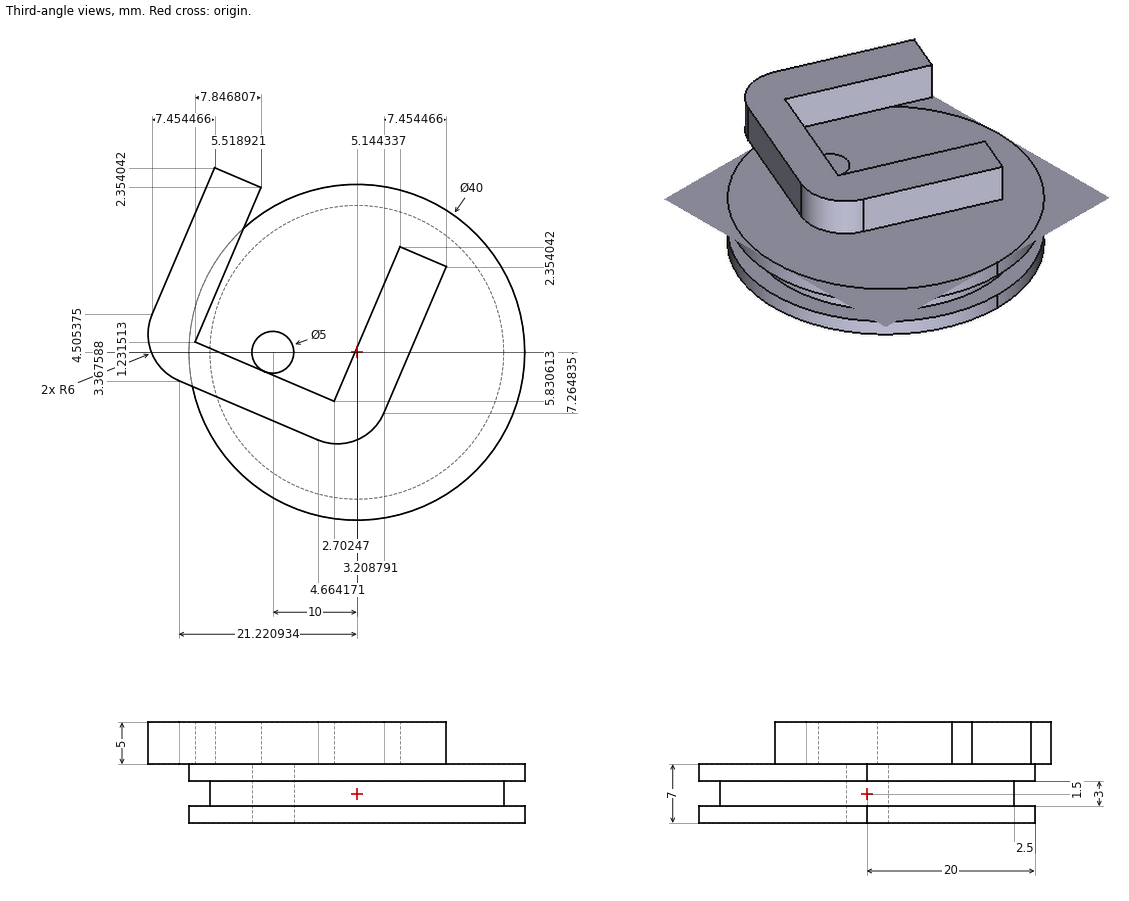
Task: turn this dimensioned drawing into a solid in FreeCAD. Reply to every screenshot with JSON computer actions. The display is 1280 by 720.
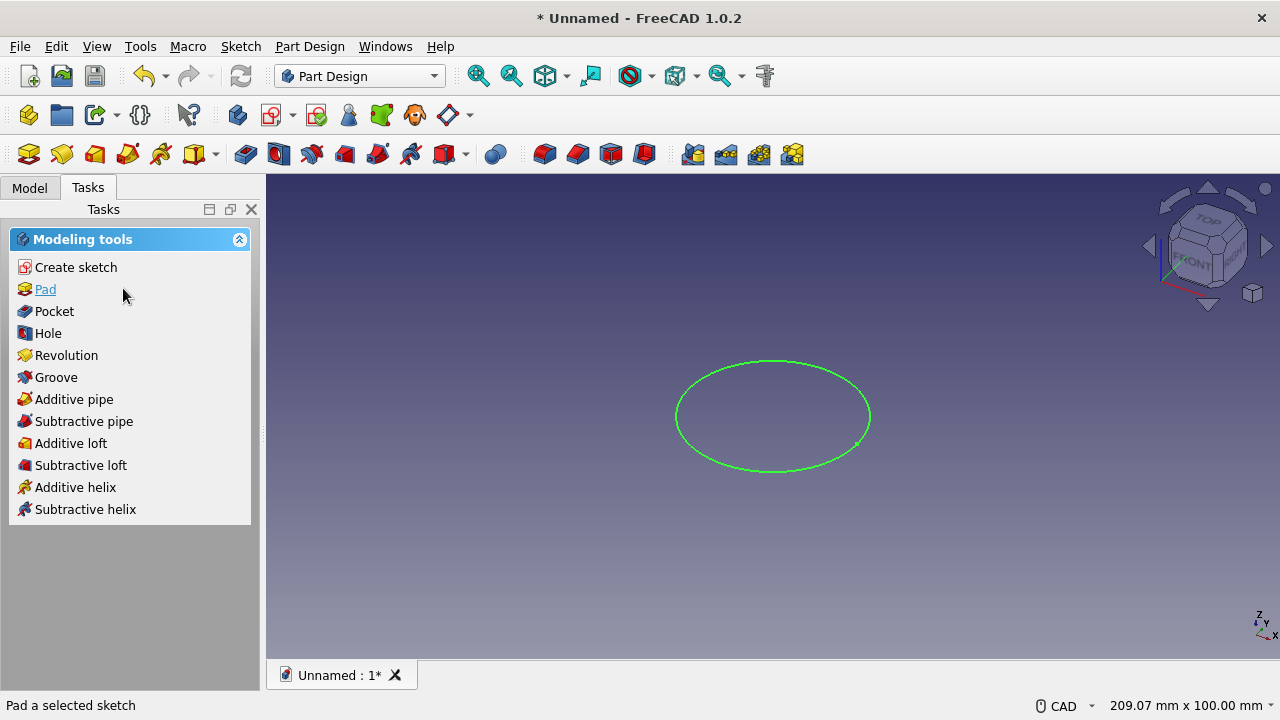
{"action": "left_click", "coordinate": [29, 154]}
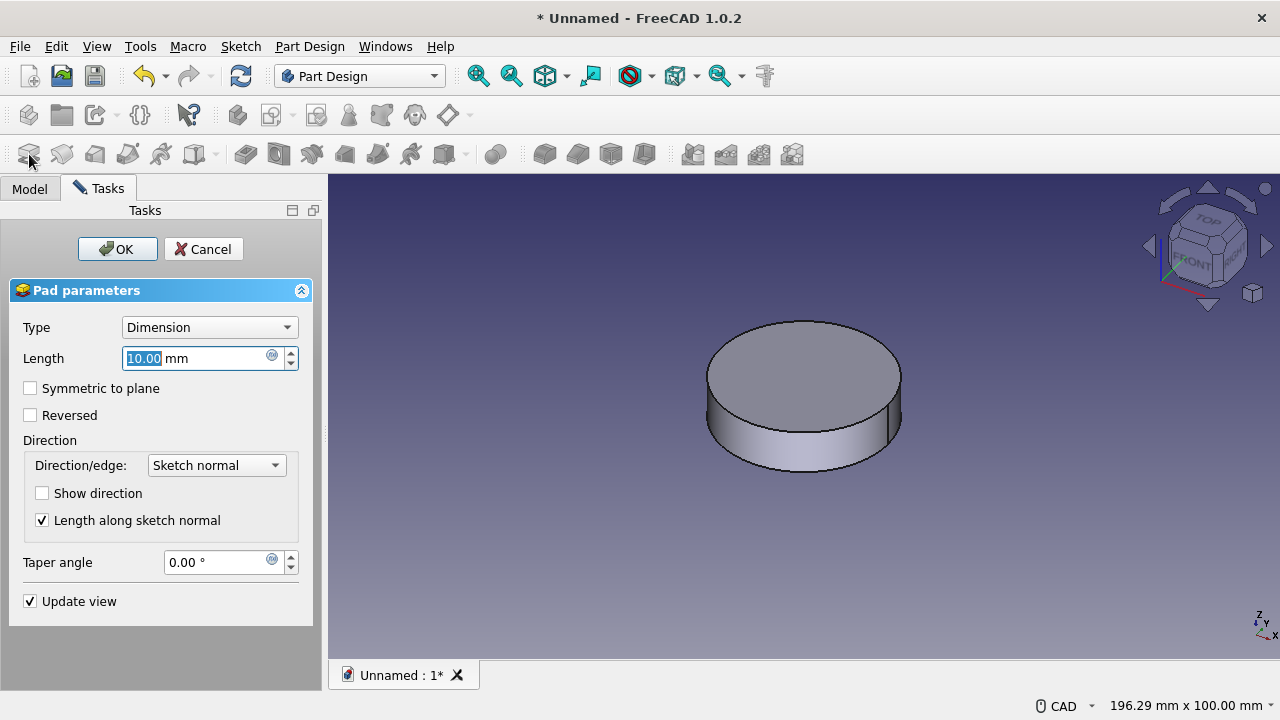
{"action": "type", "text": "7"}
{"action": "key", "text": "Tab"}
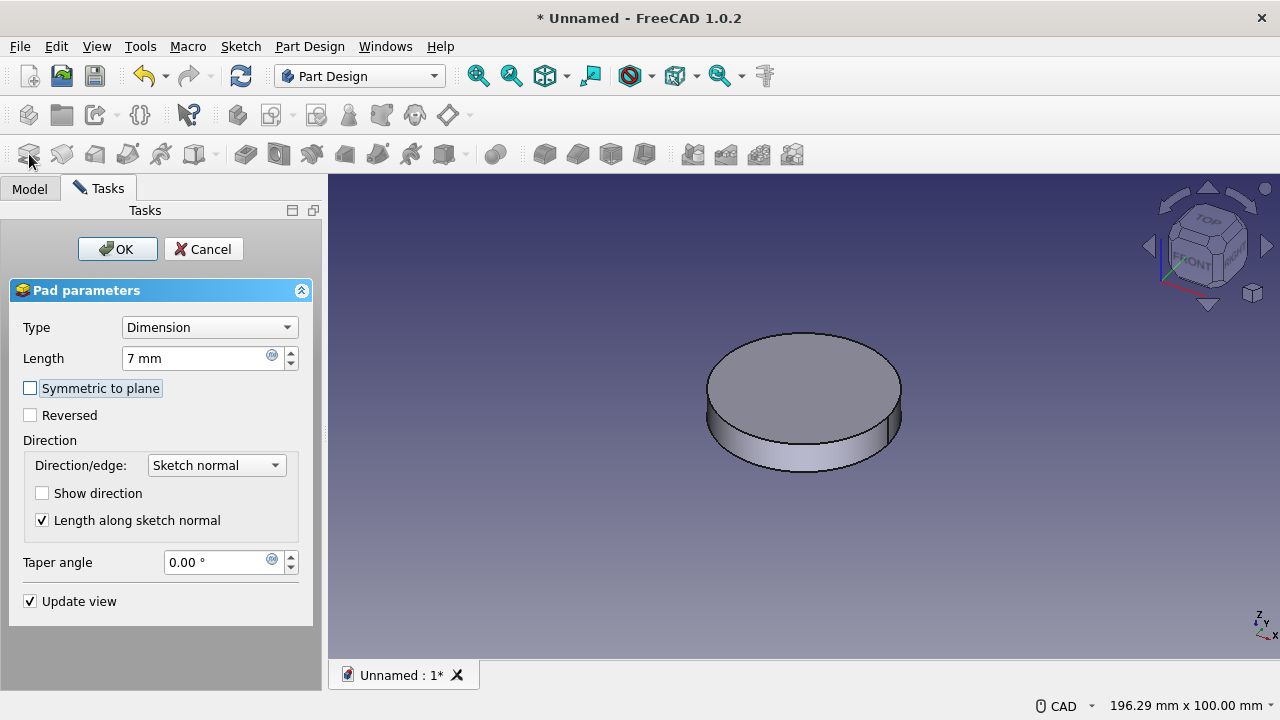
{"action": "left_click", "coordinate": [31, 388]}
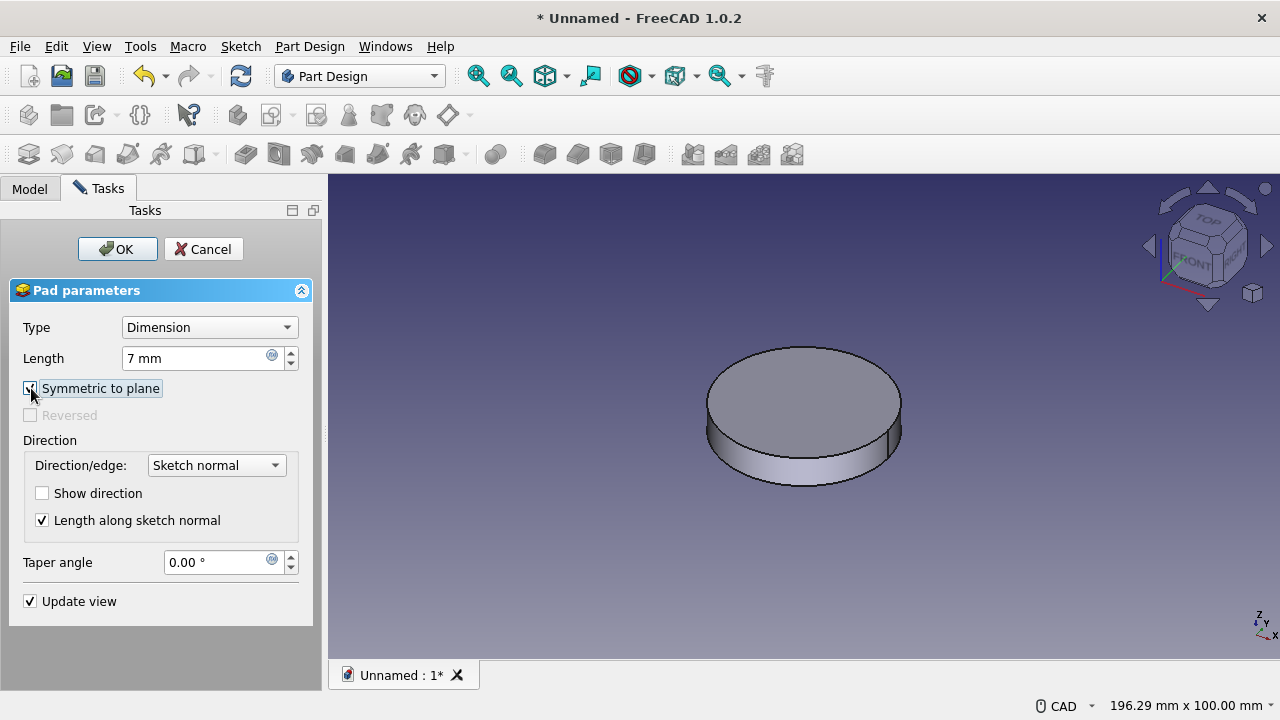
{"action": "left_click", "coordinate": [118, 249]}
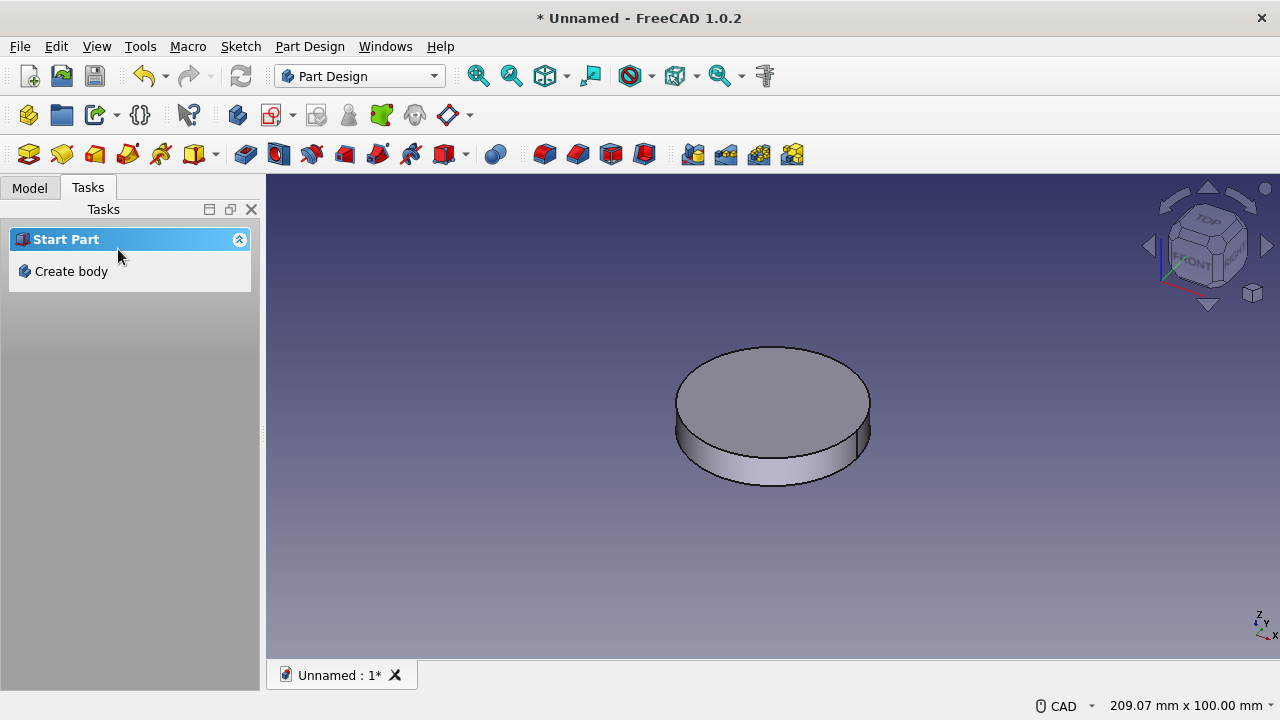
{"action": "left_click", "coordinate": [479, 76]}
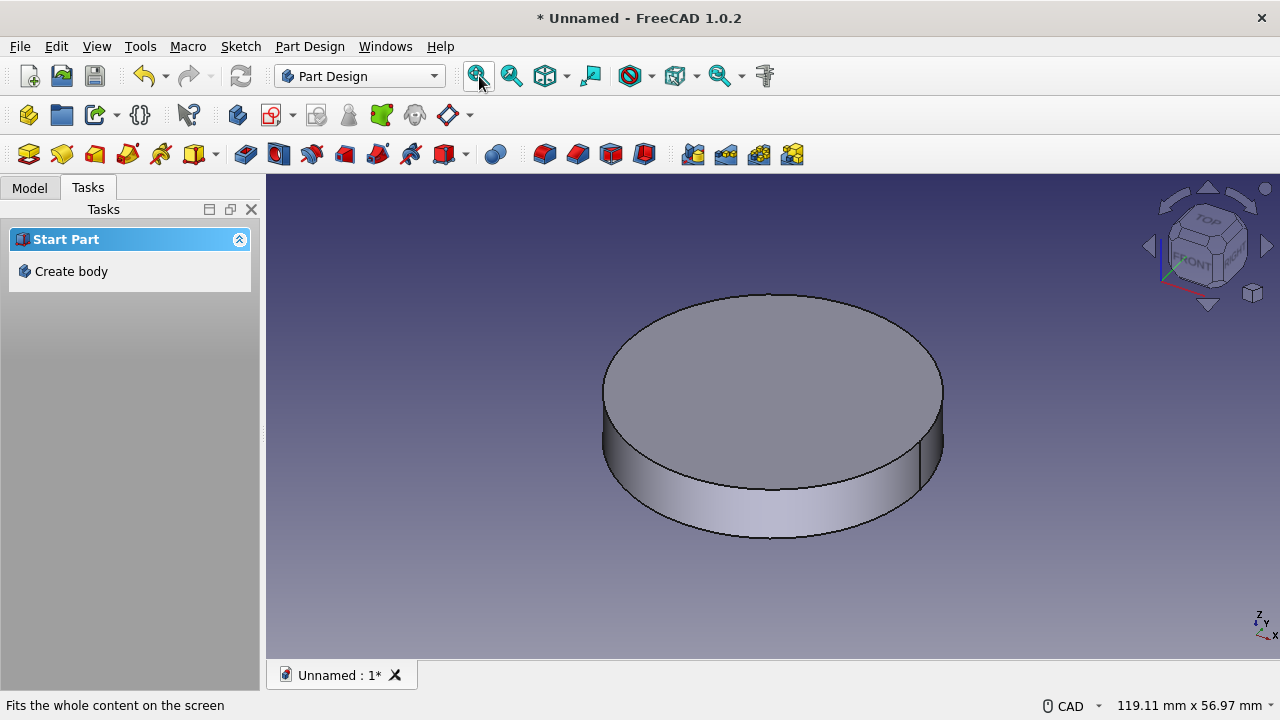
{"action": "left_click", "coordinate": [270, 116]}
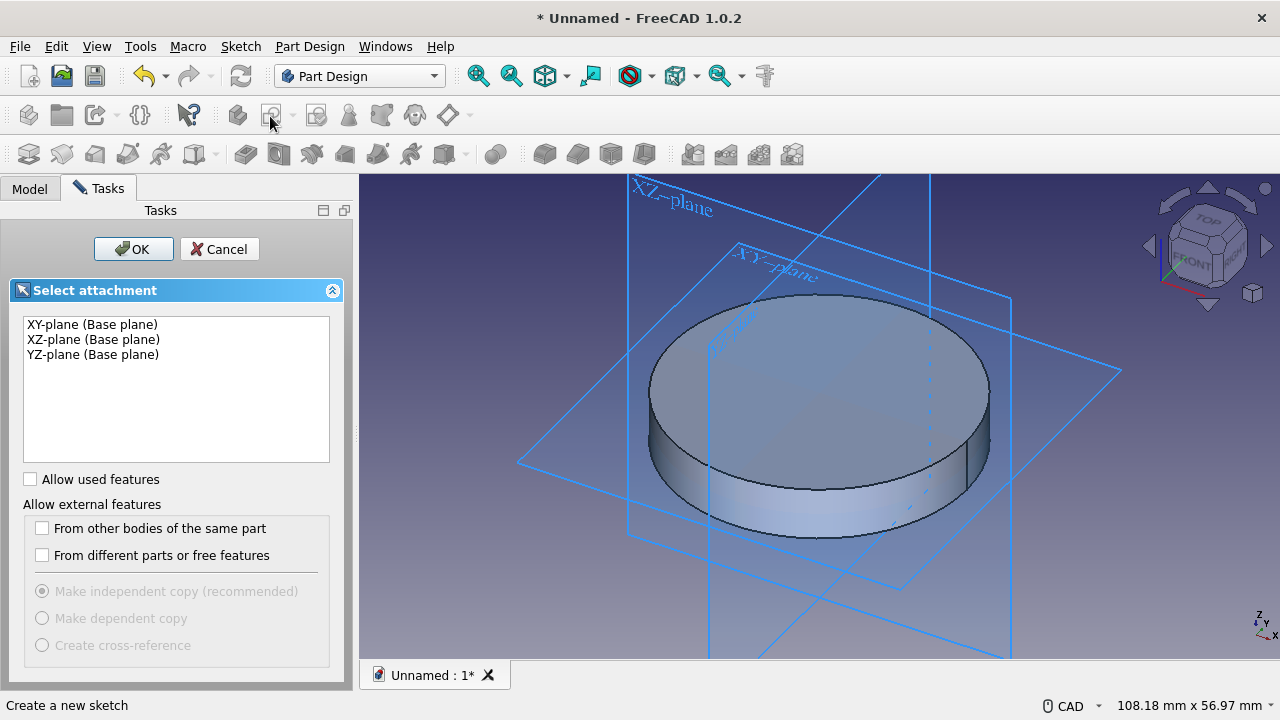
{"action": "left_click", "coordinate": [84, 354]}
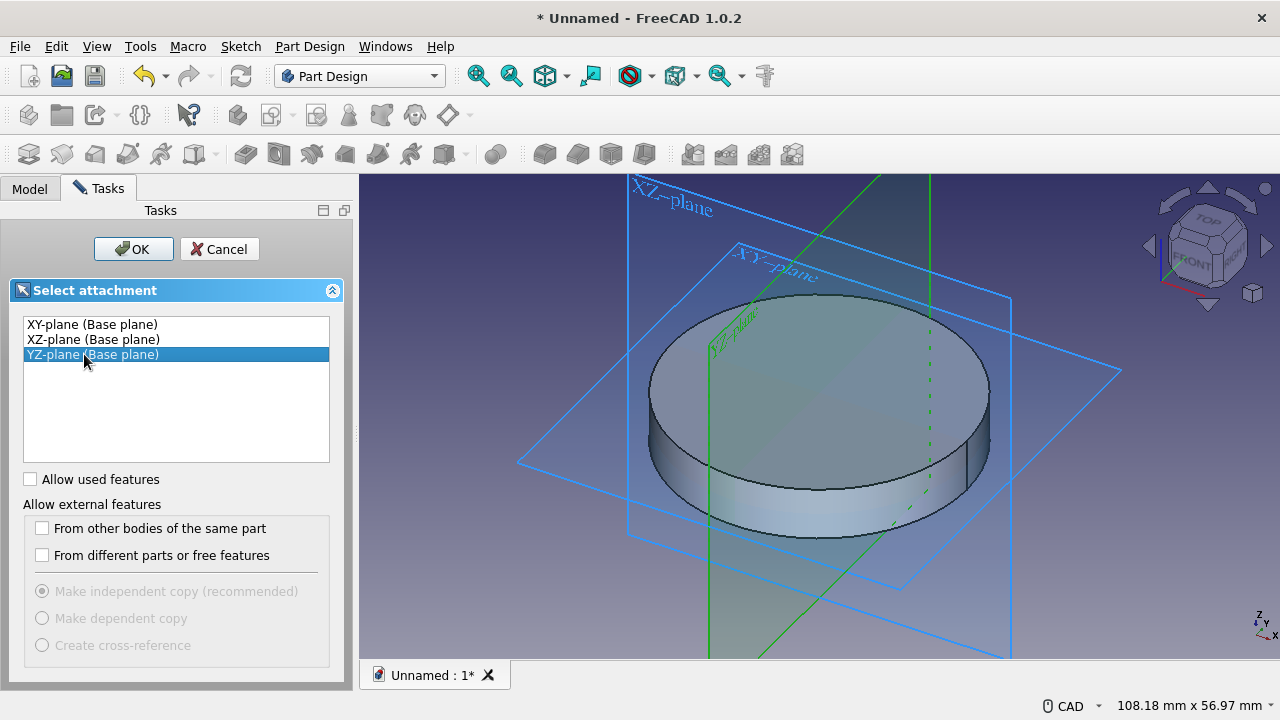
{"action": "left_click", "coordinate": [134, 249]}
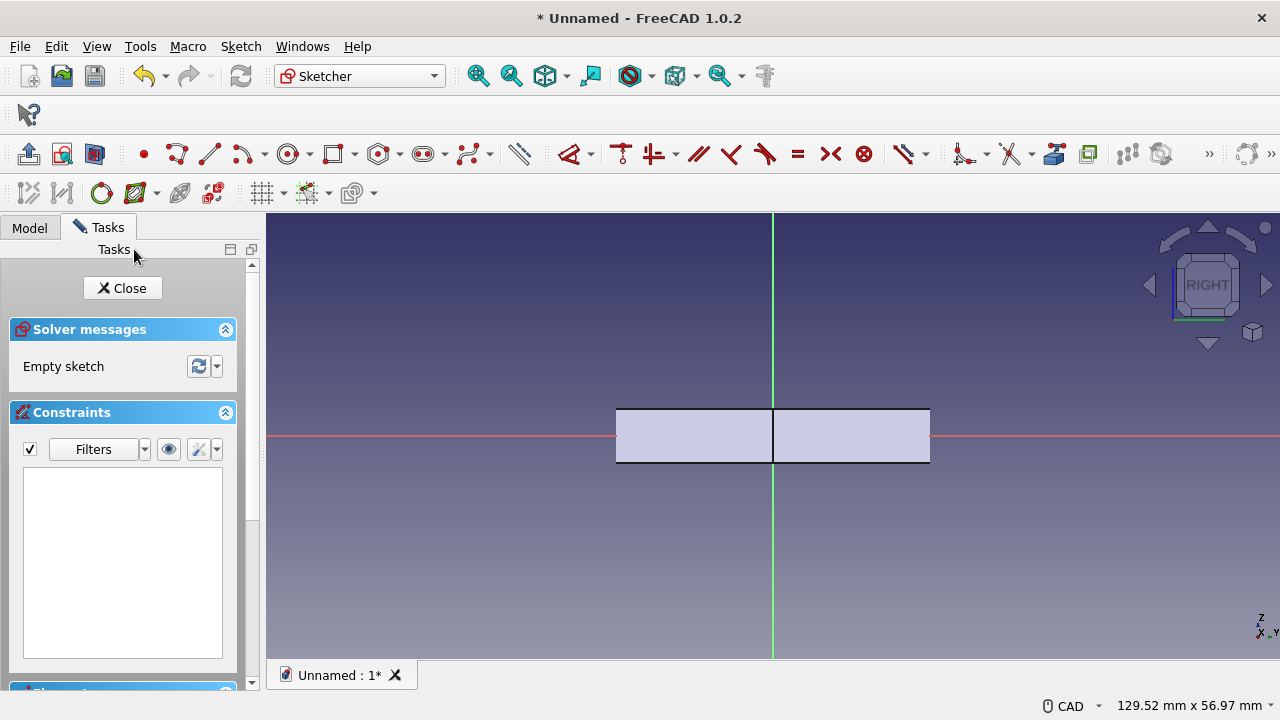
{"action": "left_click", "coordinate": [95, 154]}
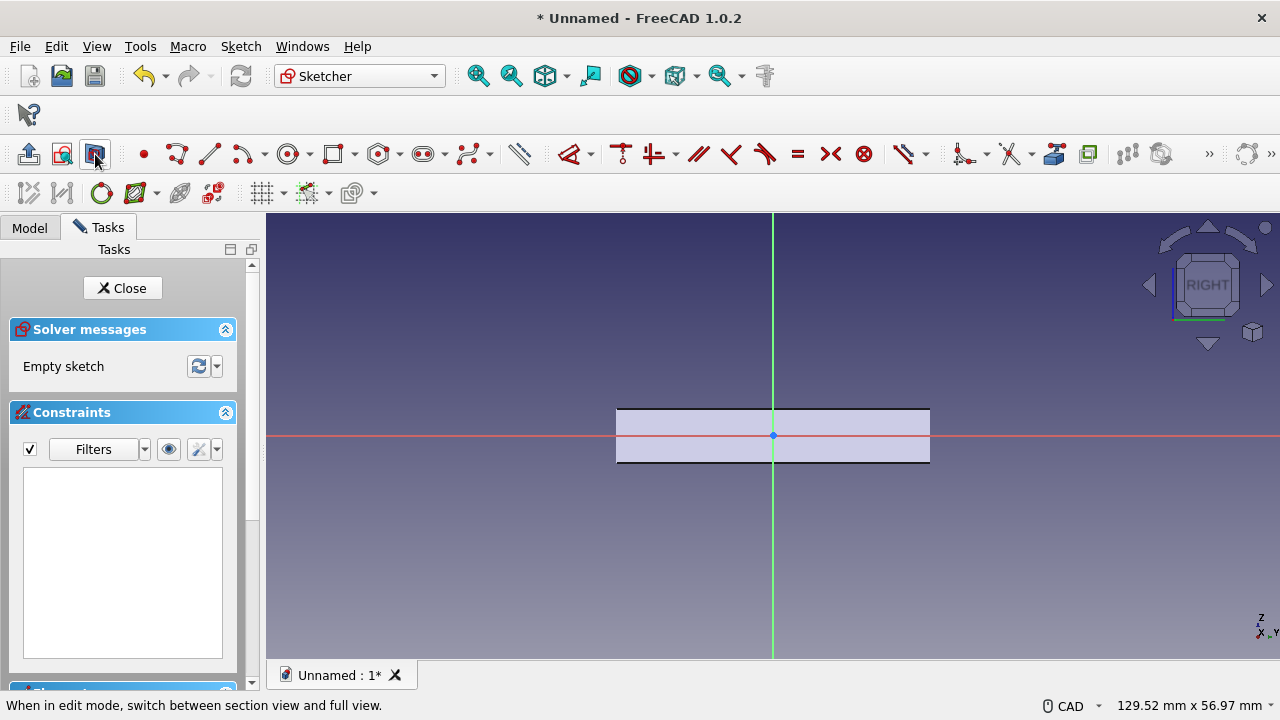
{"action": "scroll", "coordinate": [941, 436], "scroll_direction": "up", "scroll_amount": 12}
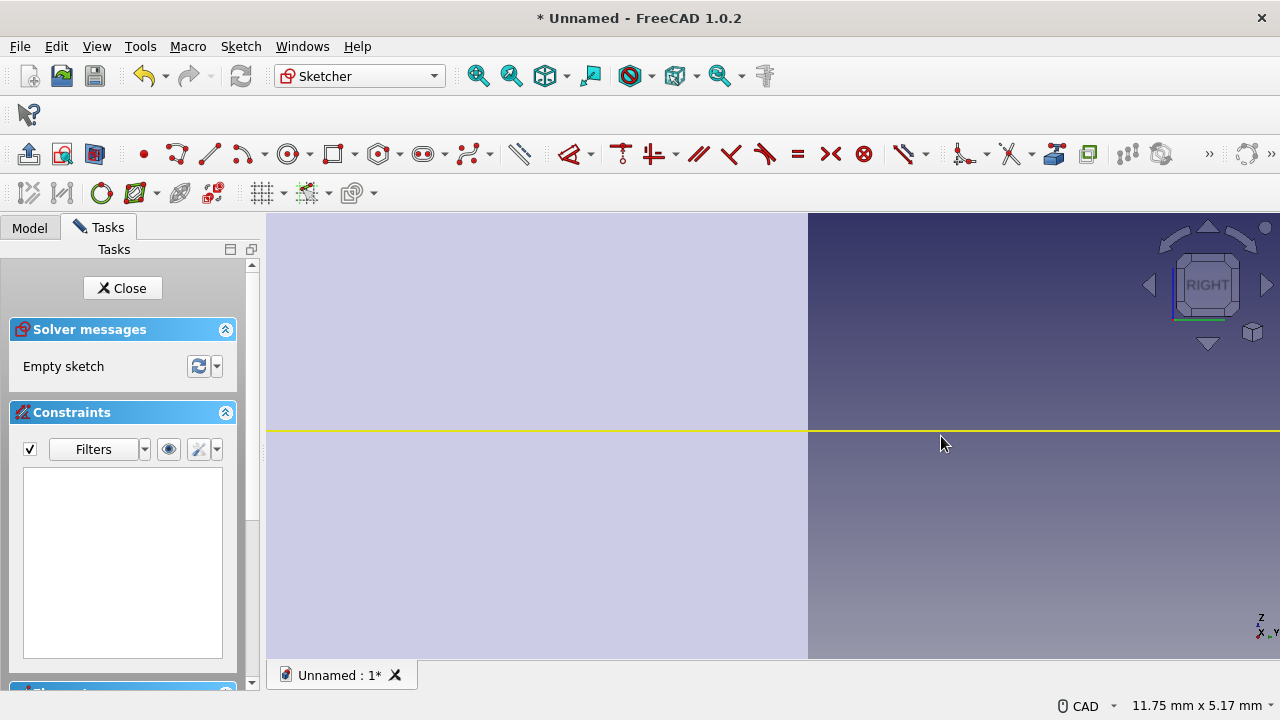
{"action": "left_click", "coordinate": [332, 154]}